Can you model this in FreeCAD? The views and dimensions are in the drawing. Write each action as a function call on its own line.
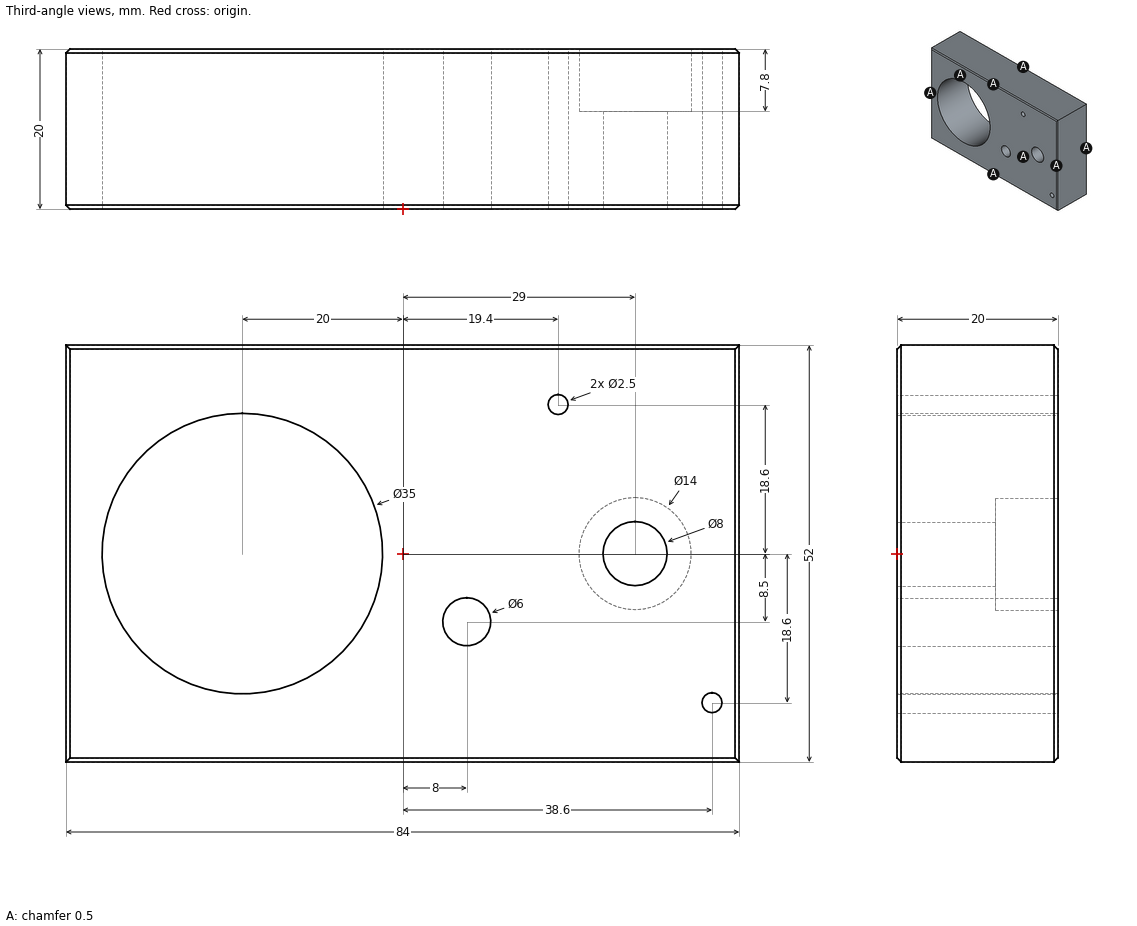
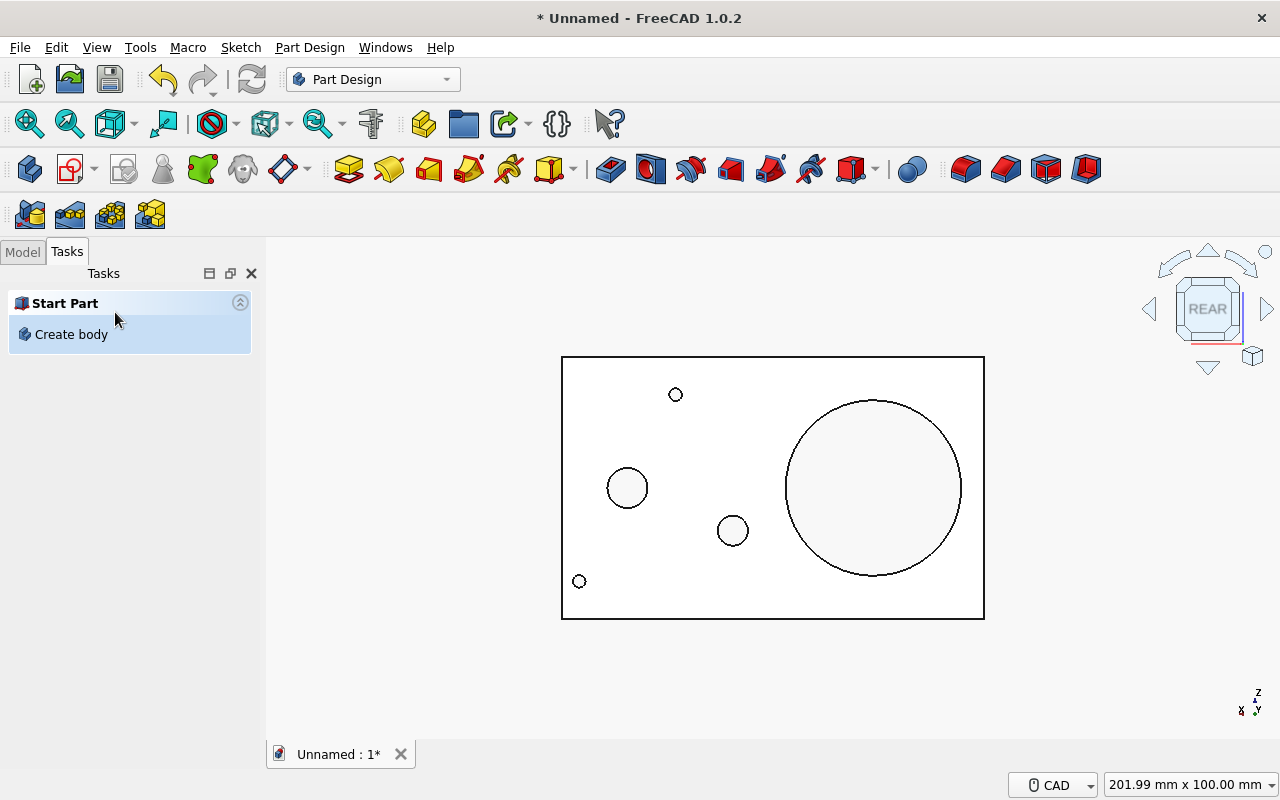
click(713, 450)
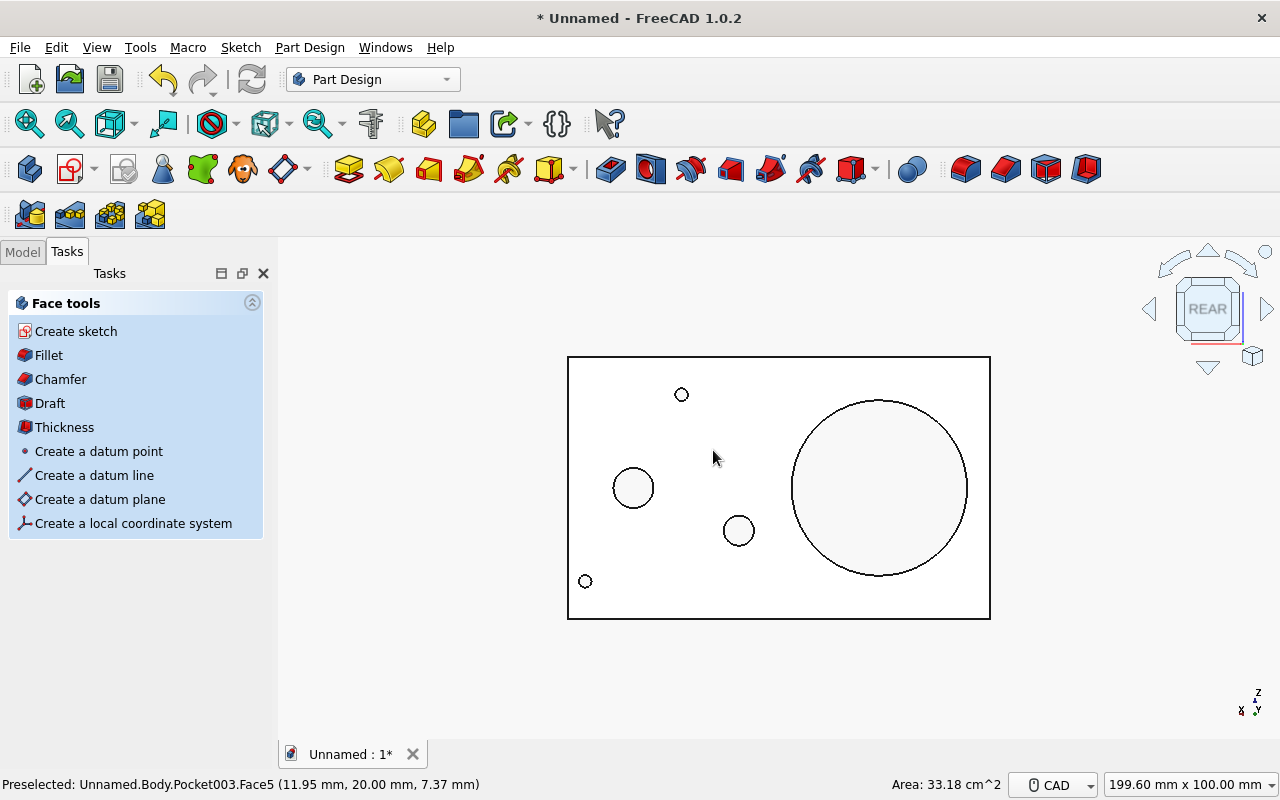
click(70, 170)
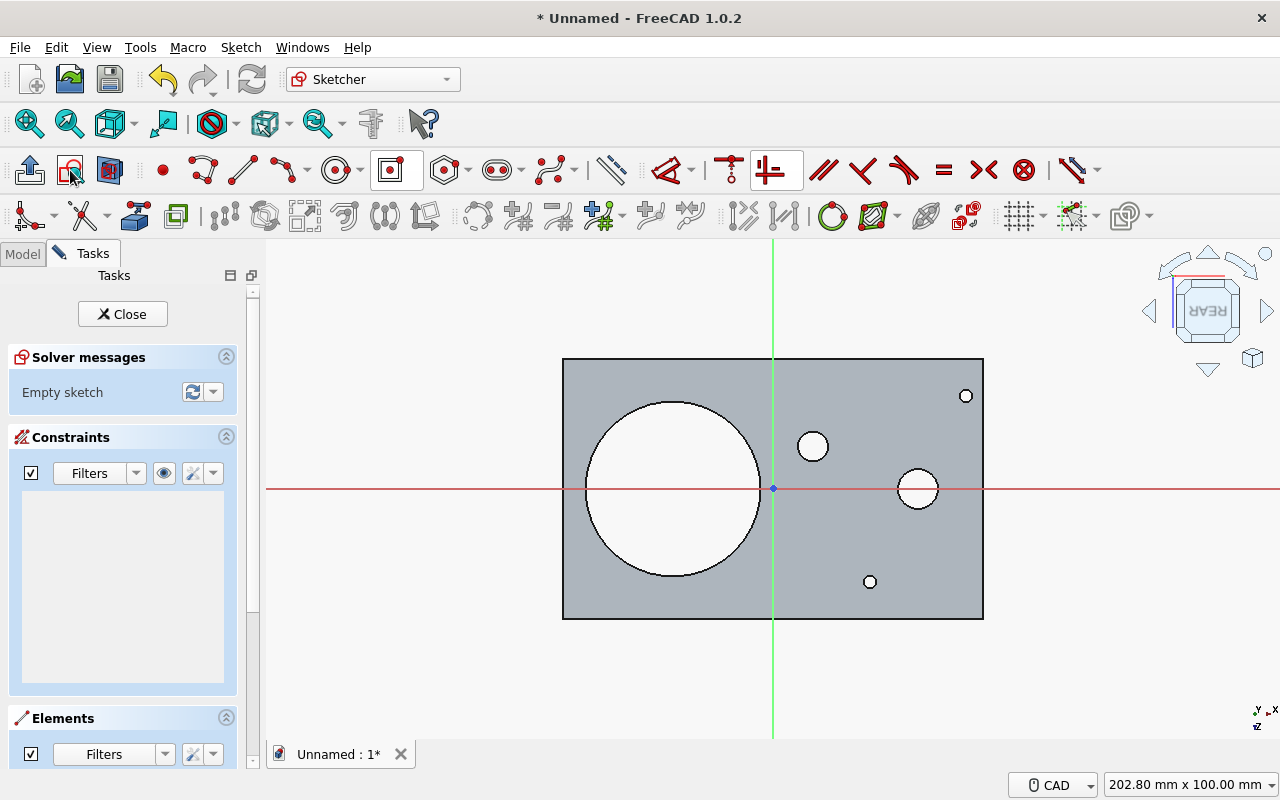
scroll(988, 489, up, 7)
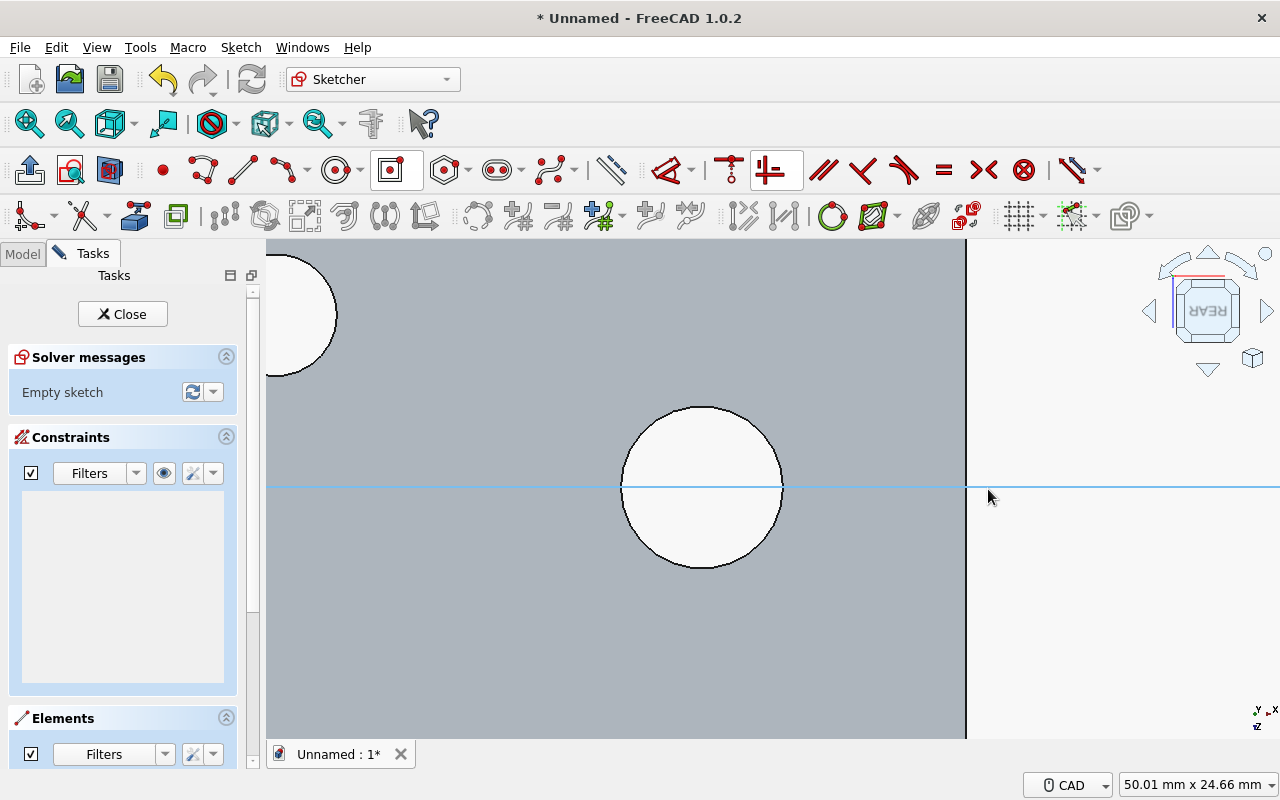
click(336, 170)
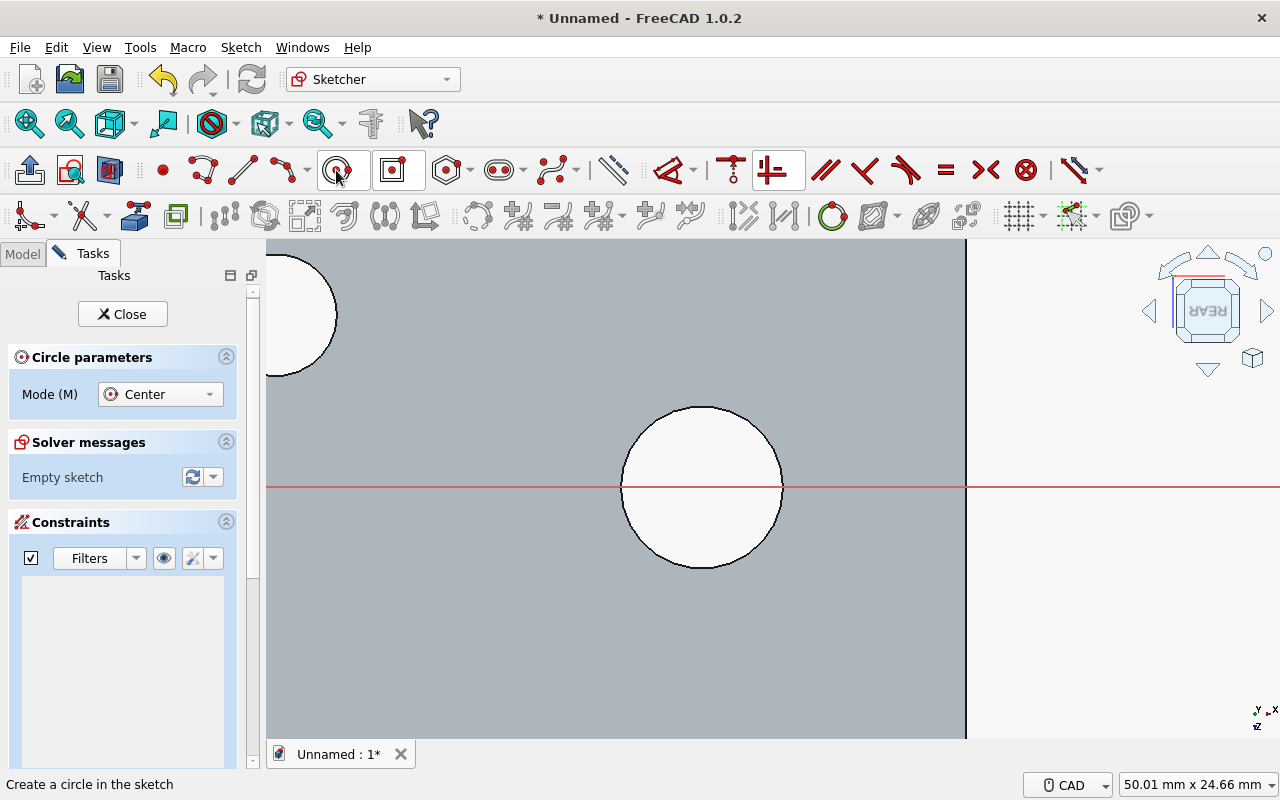
click(702, 487)
move(802, 387)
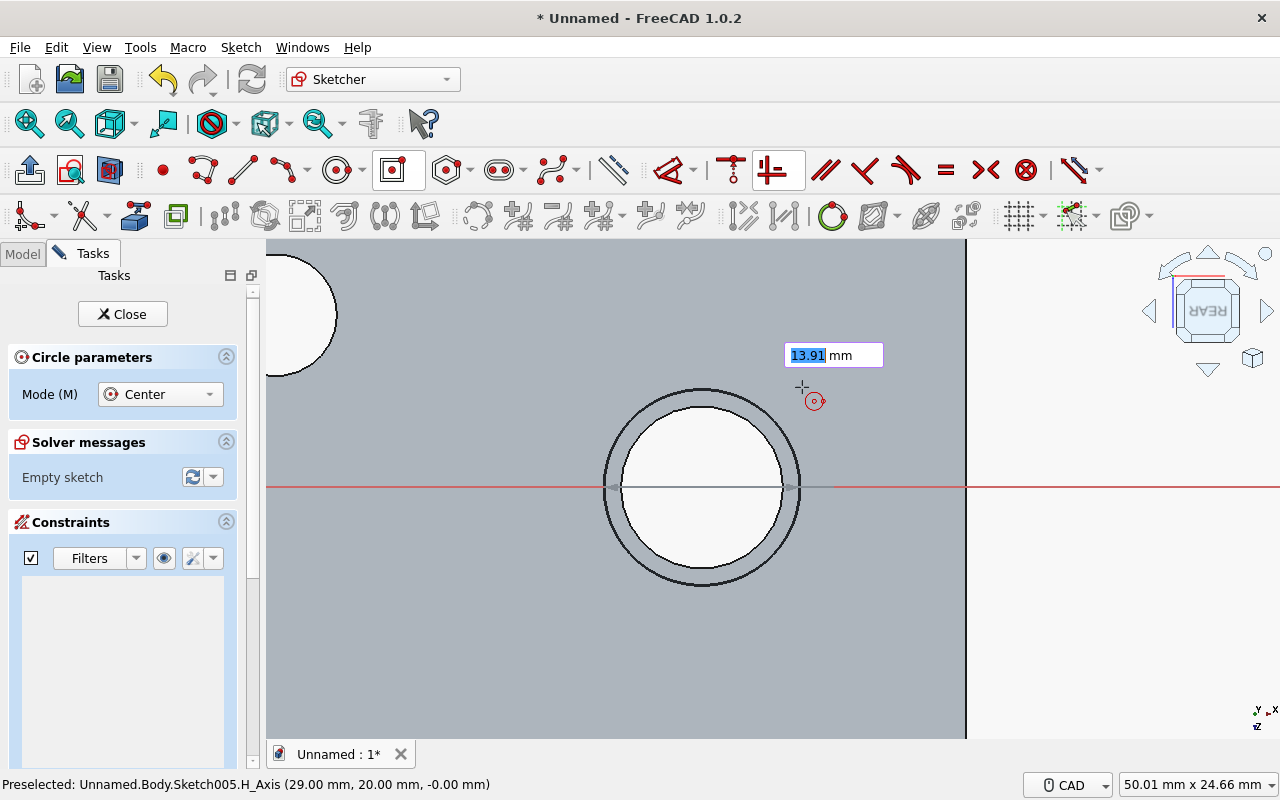
text(14)
key(Return)
key(Escape)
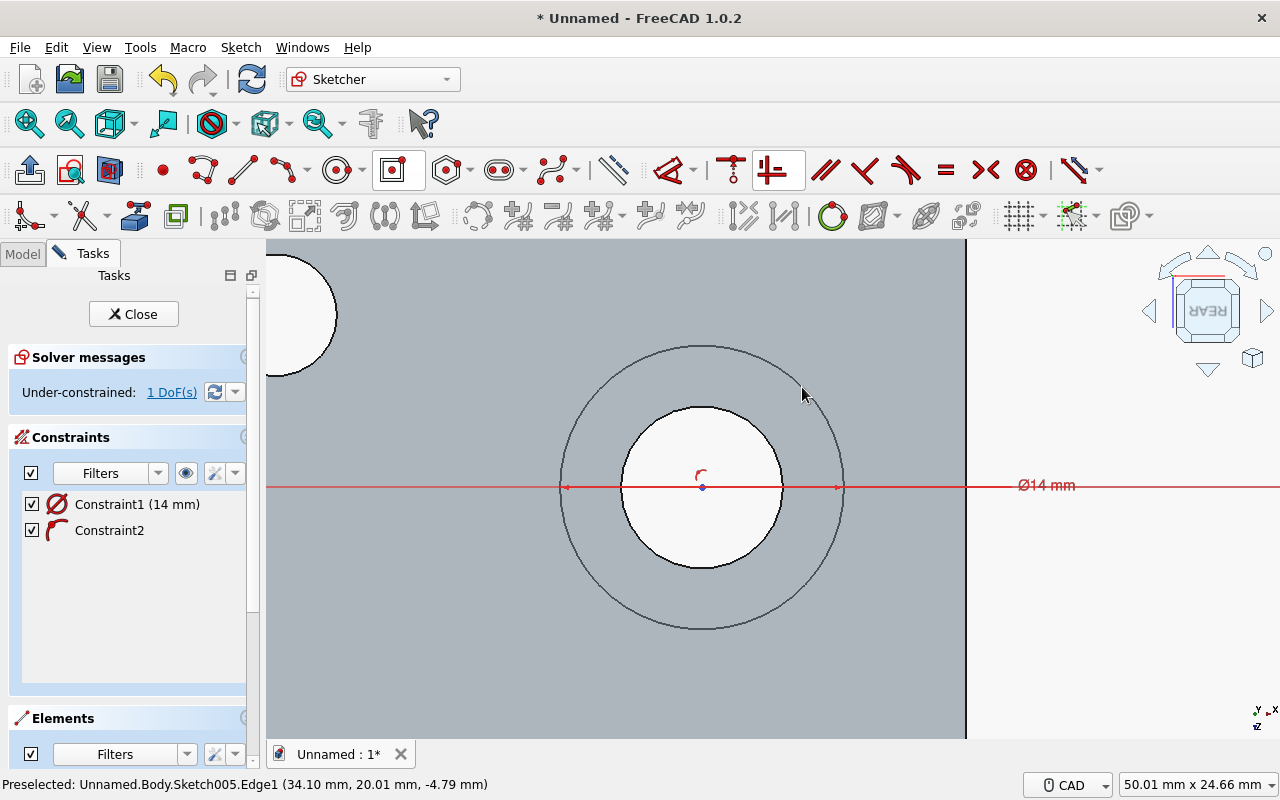
click(668, 170)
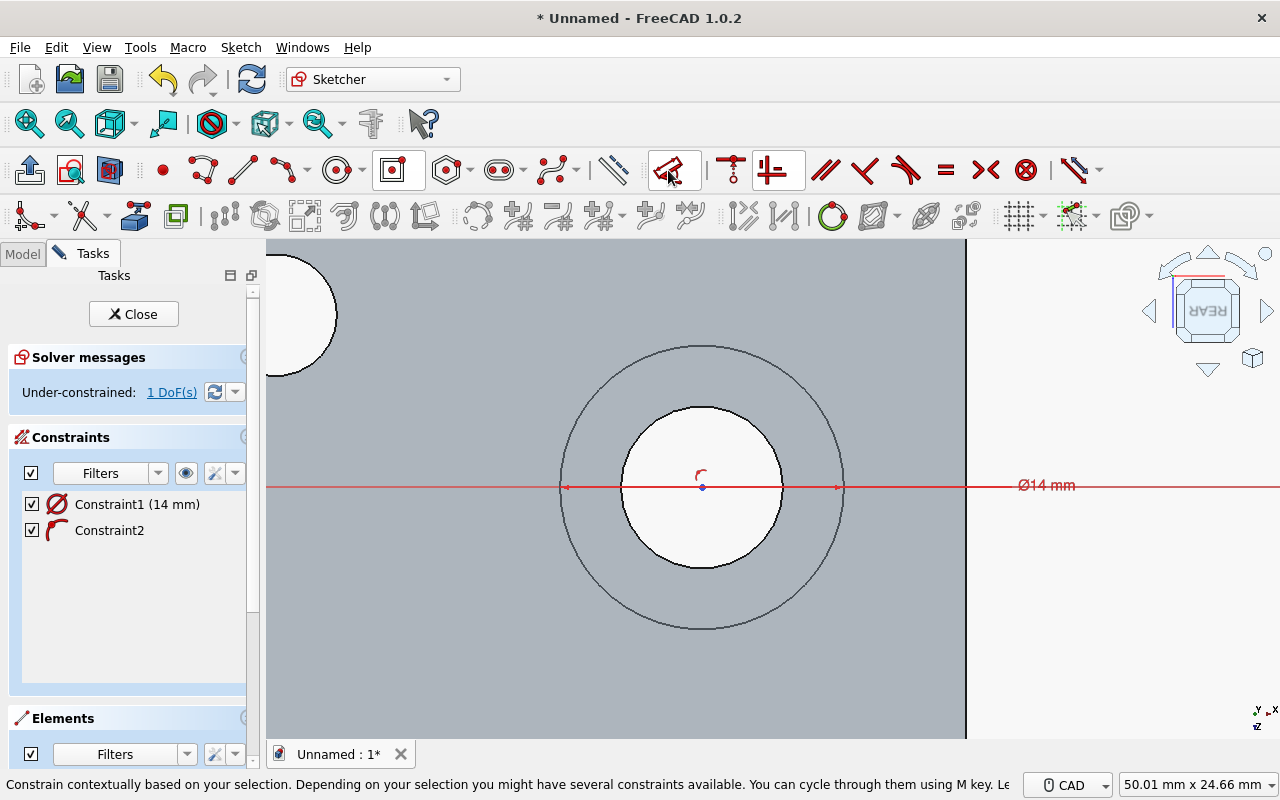
click(702, 487)
click(498, 521)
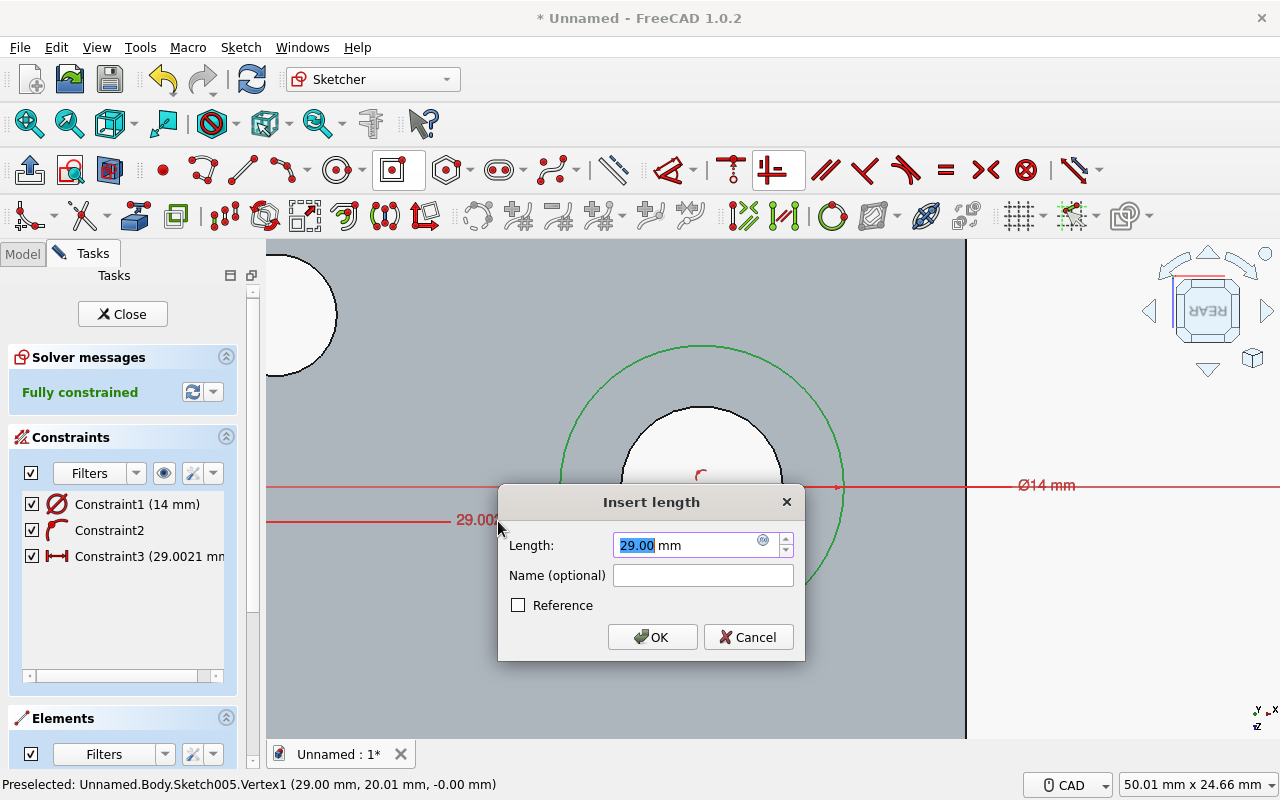
text(29)
key(Return)
key(Escape)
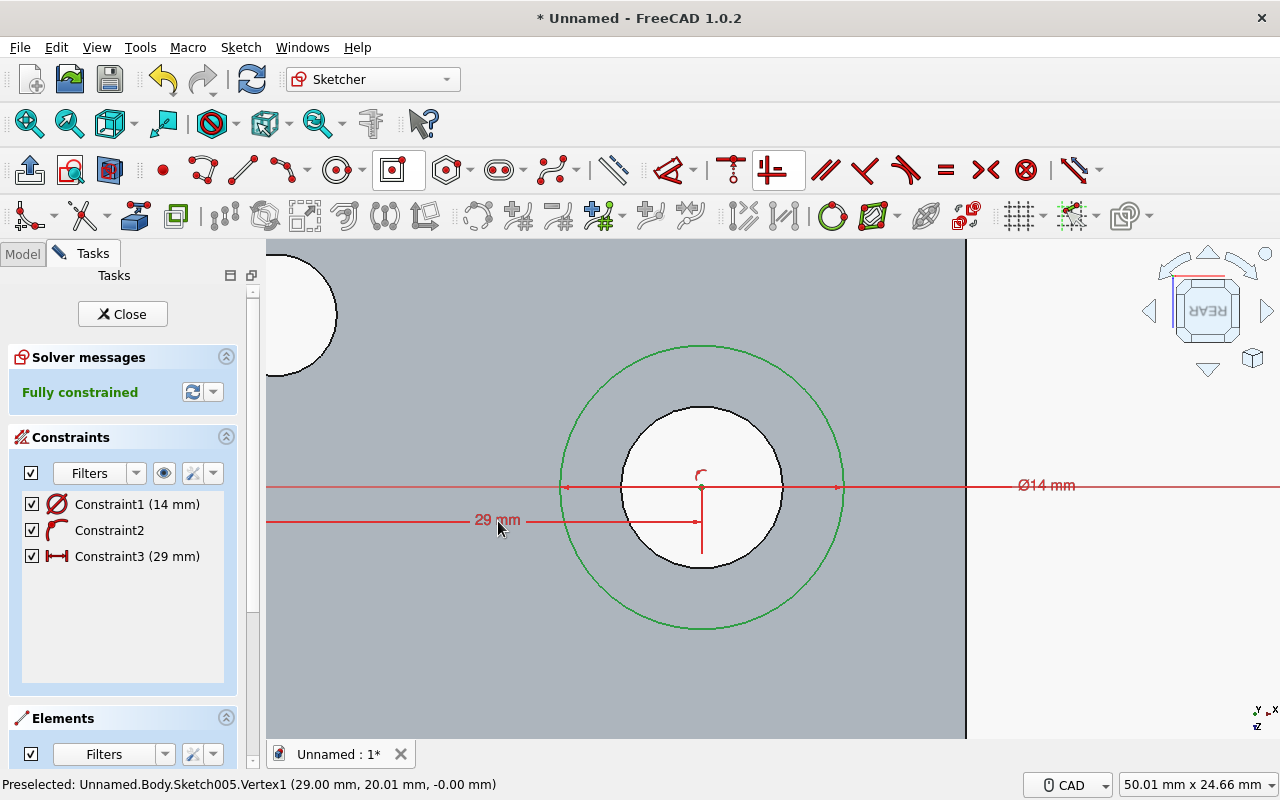
click(123, 314)